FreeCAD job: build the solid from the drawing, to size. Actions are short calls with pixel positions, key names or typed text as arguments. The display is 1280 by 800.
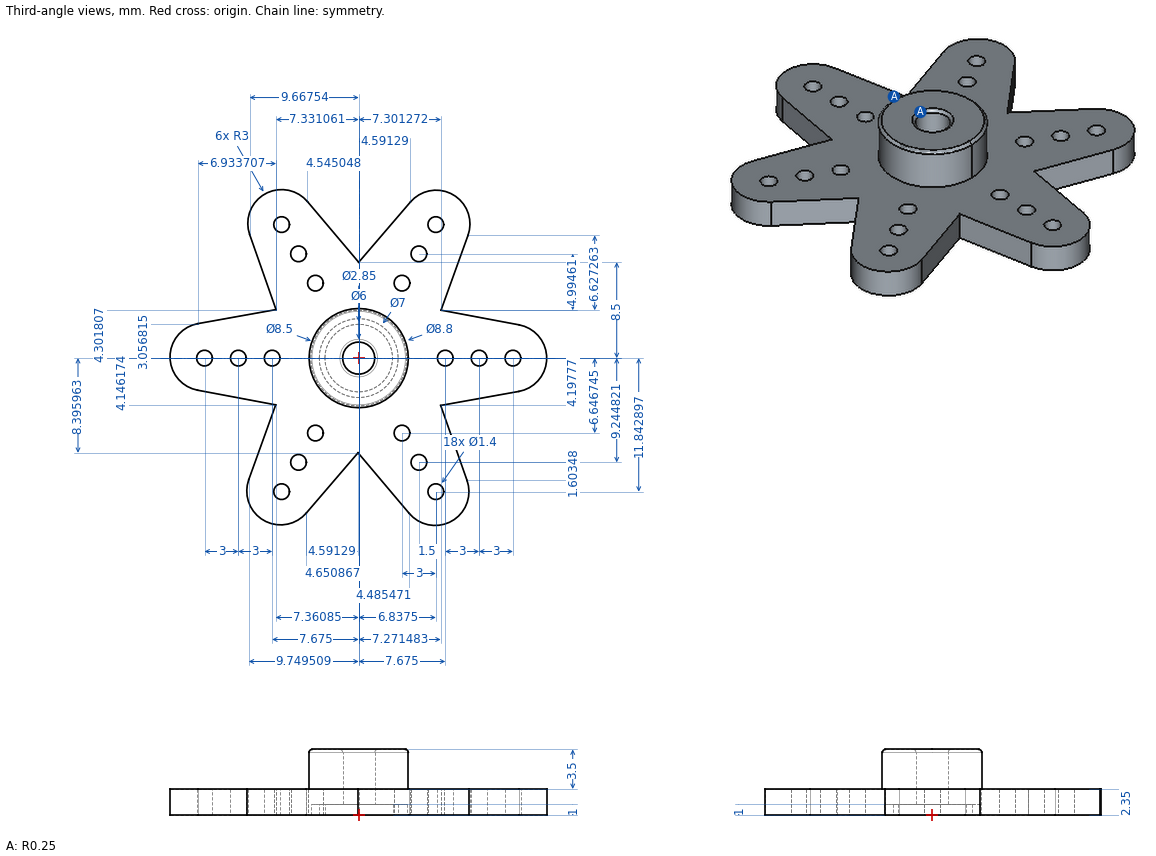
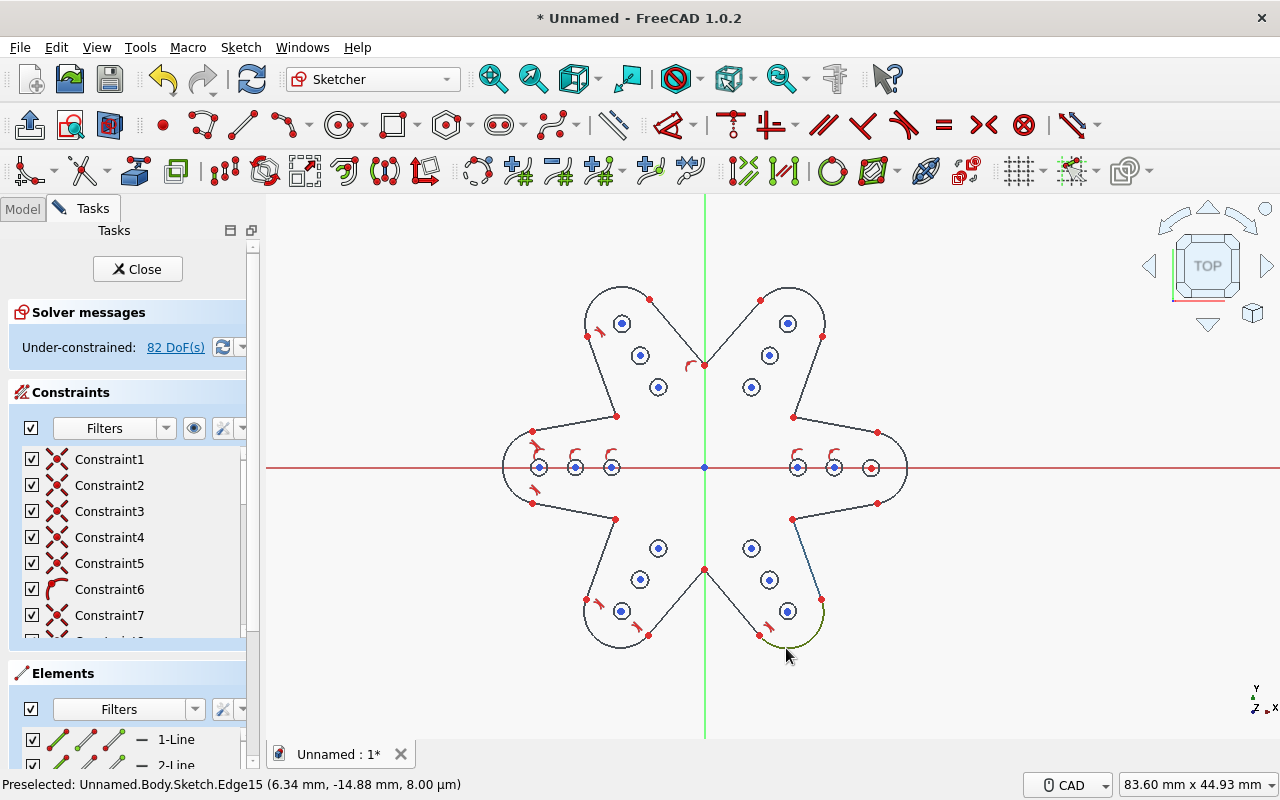
click(904, 126)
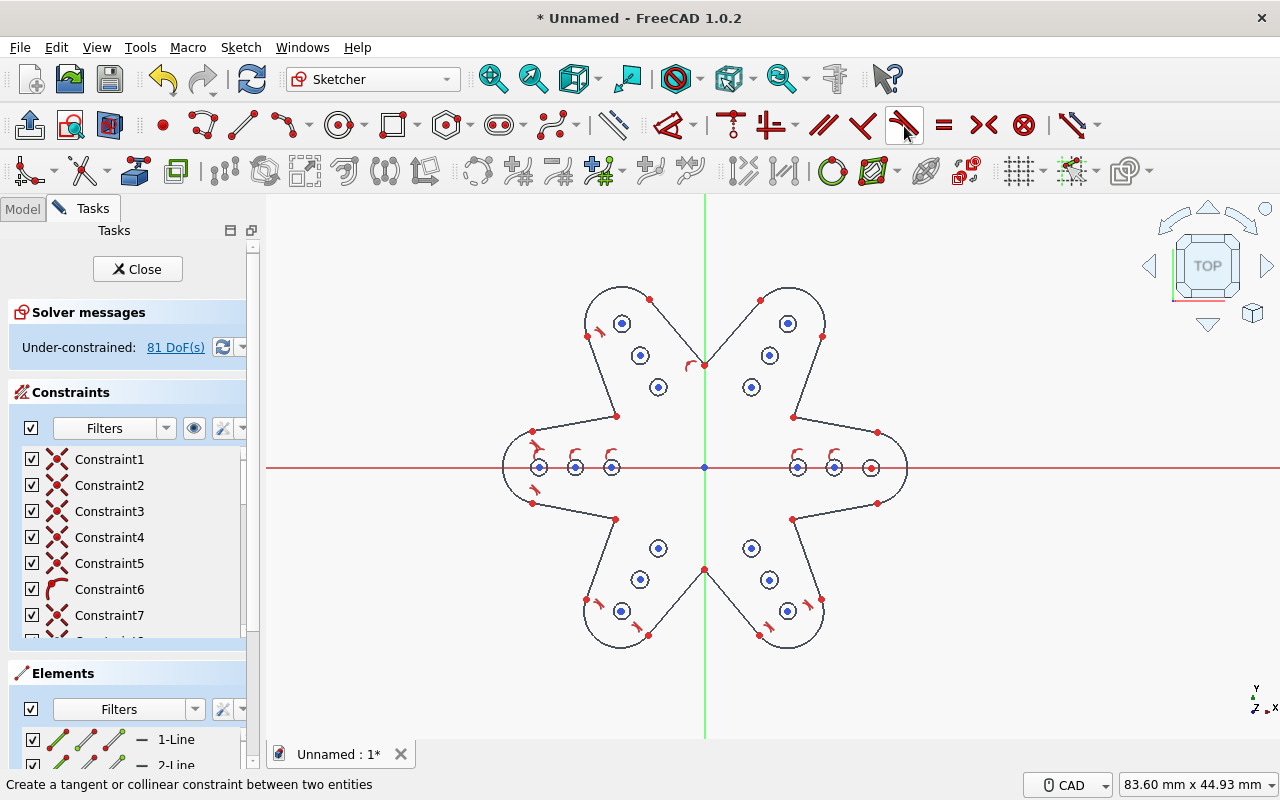
click(818, 515)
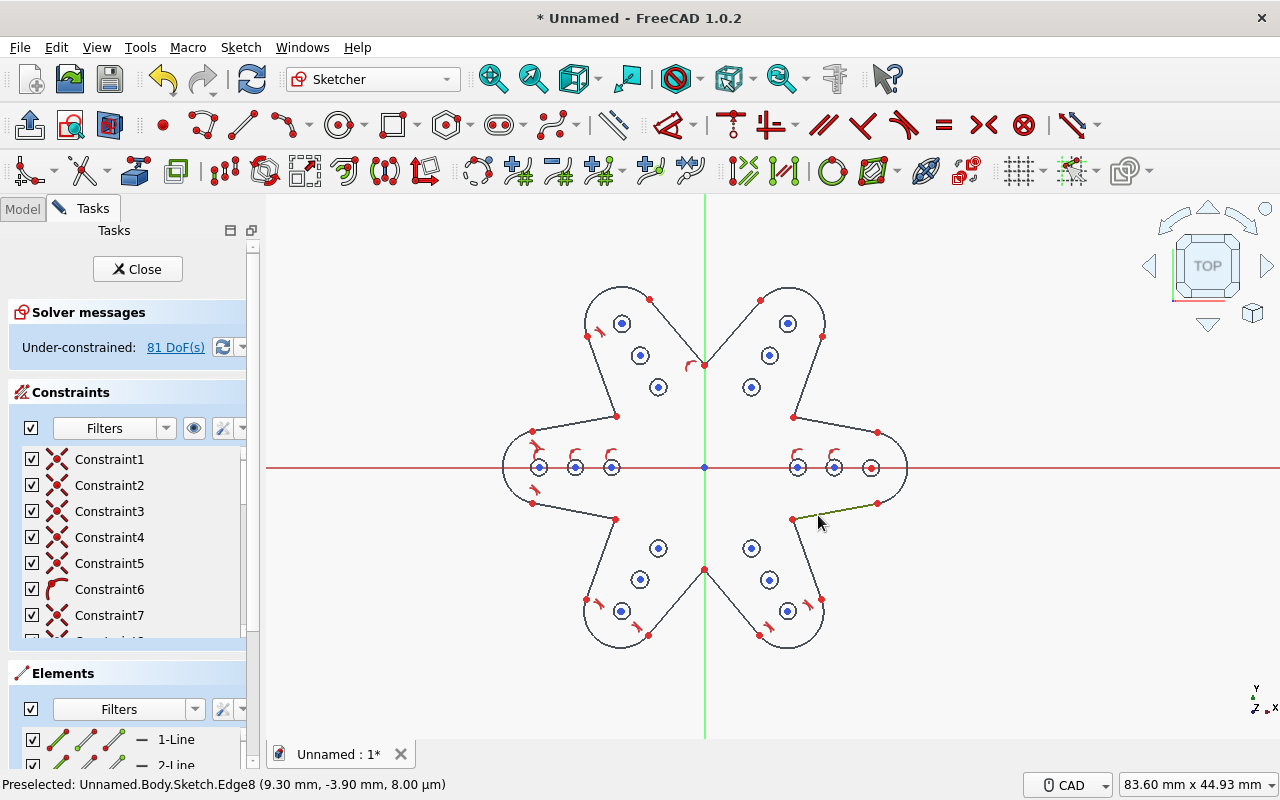
click(902, 487)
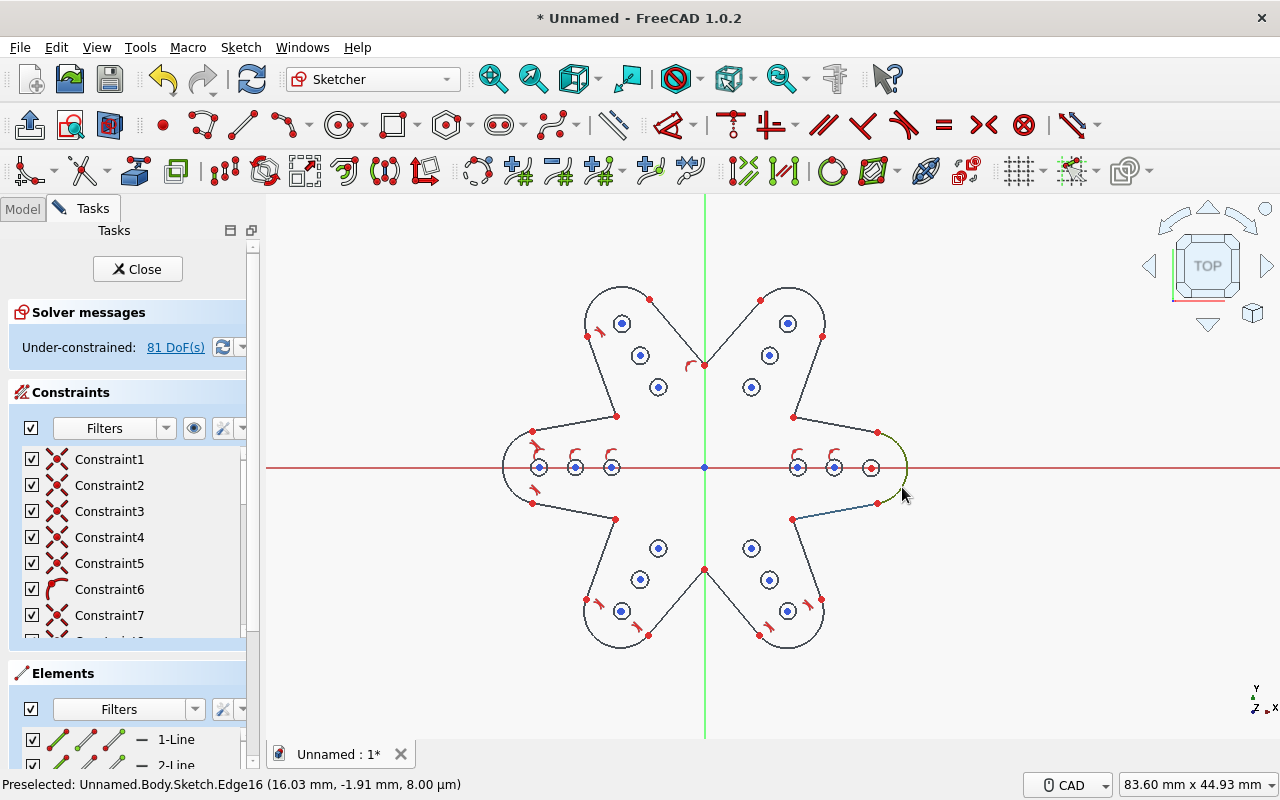
click(904, 126)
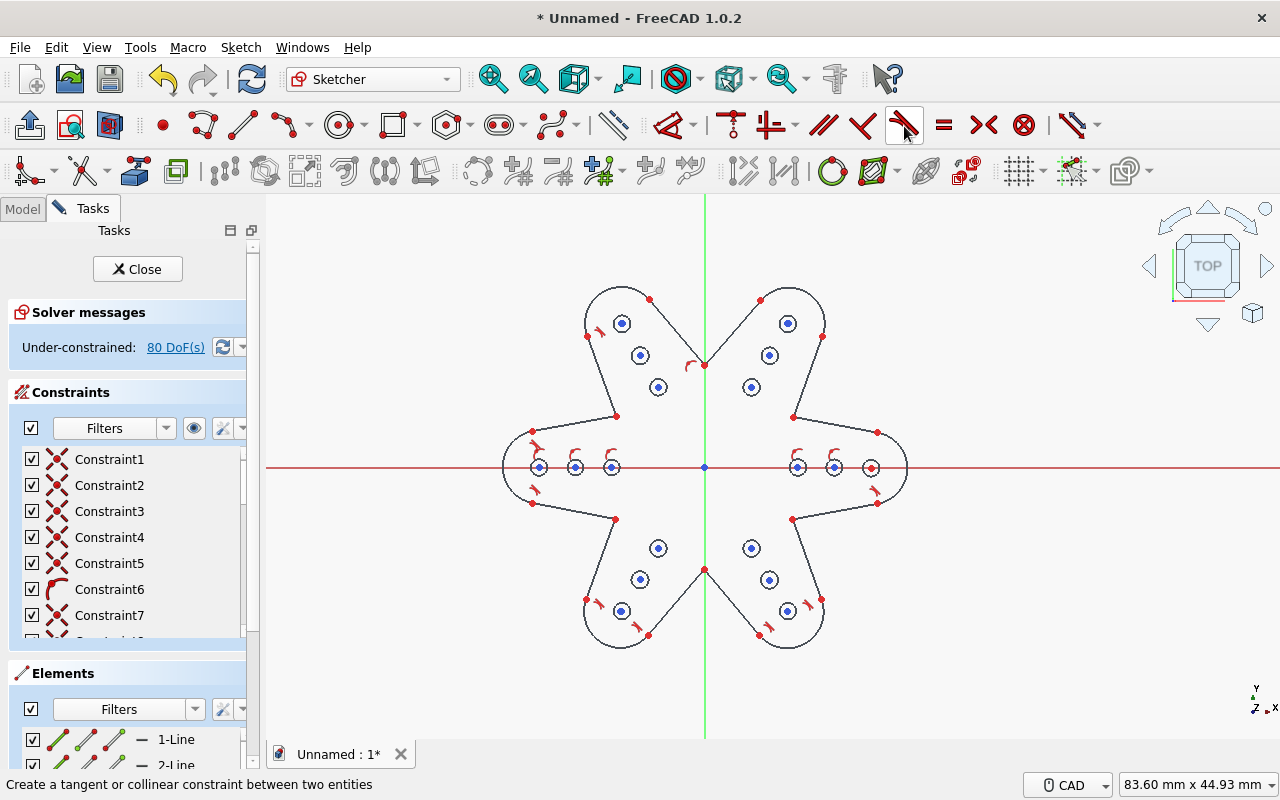
click(852, 428)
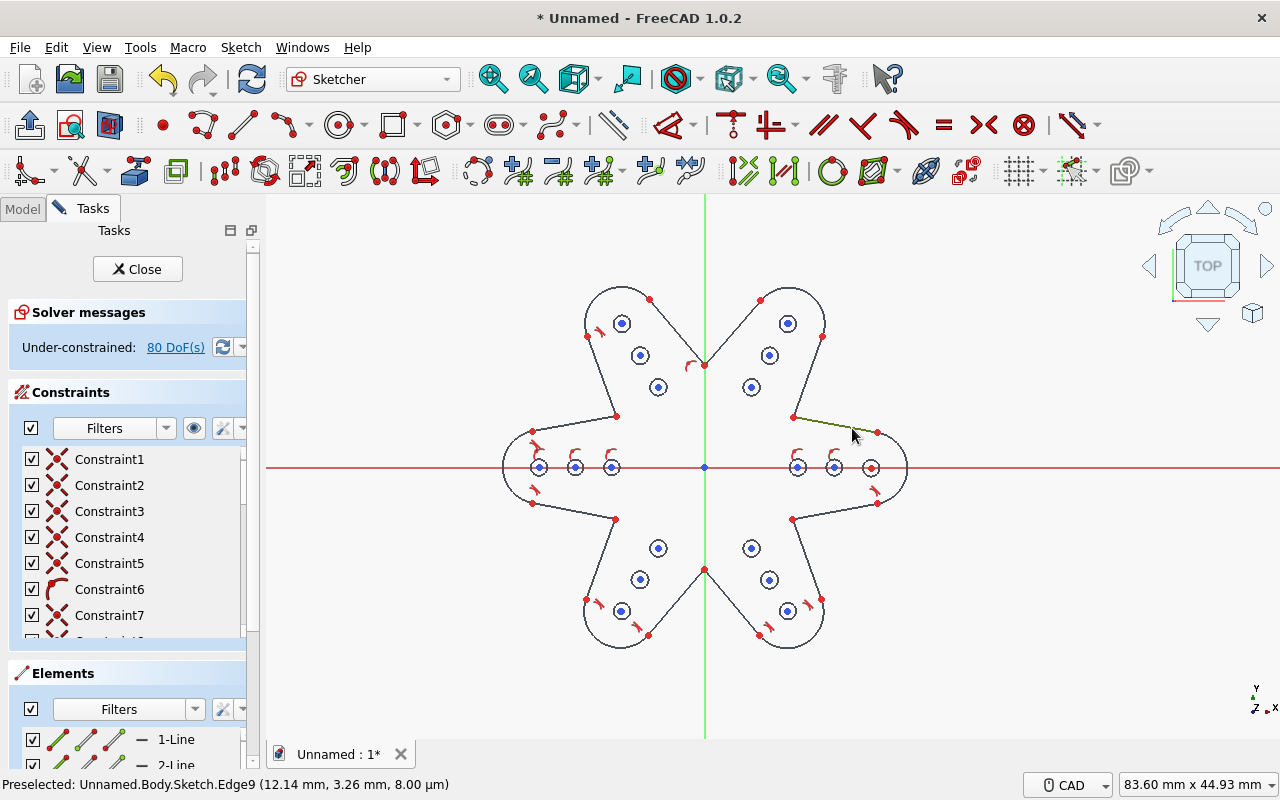
click(902, 487)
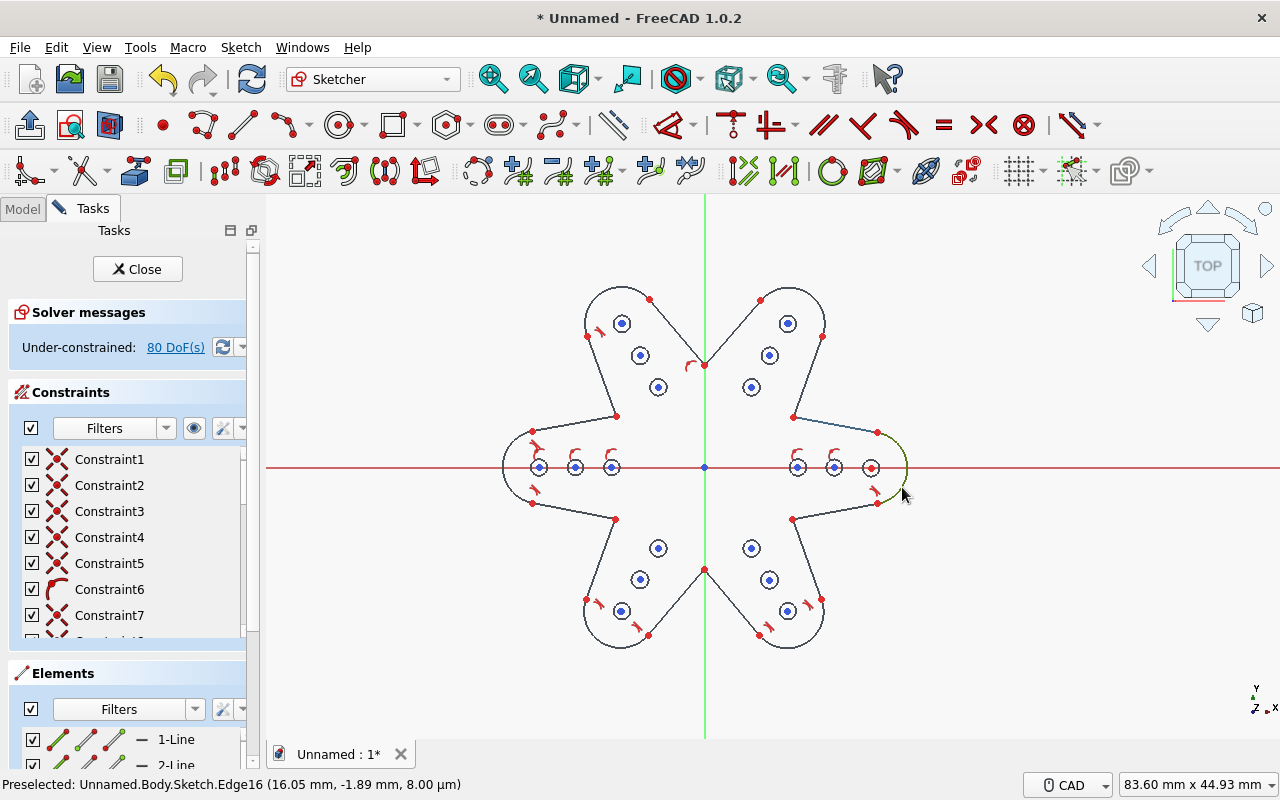
click(904, 126)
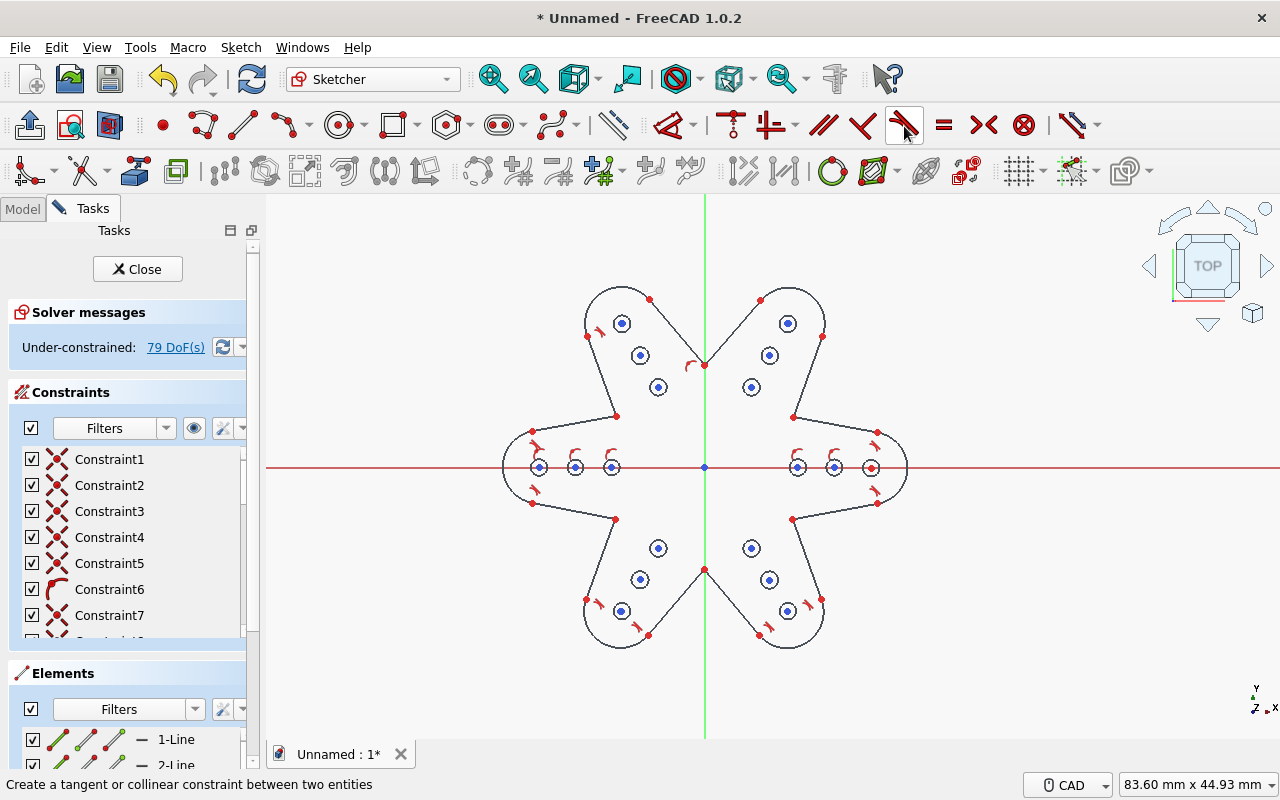
click(802, 393)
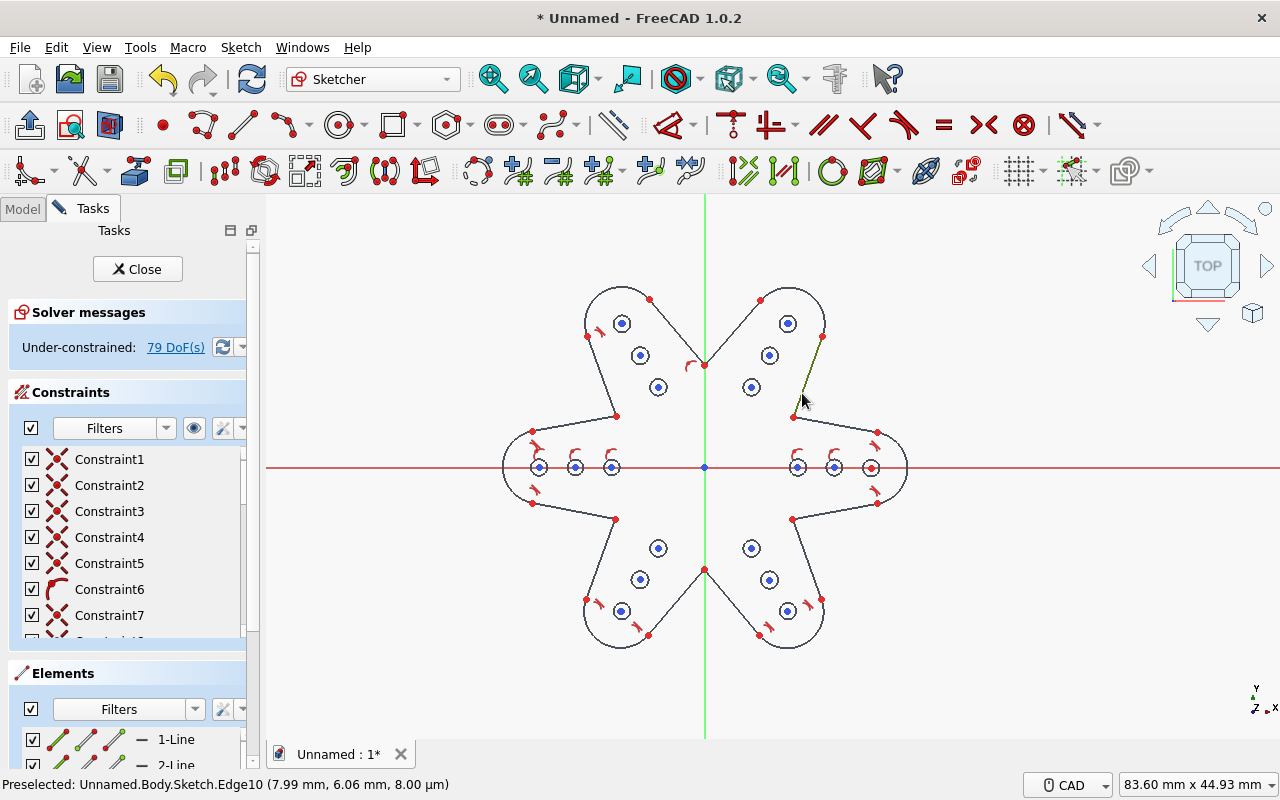
click(821, 307)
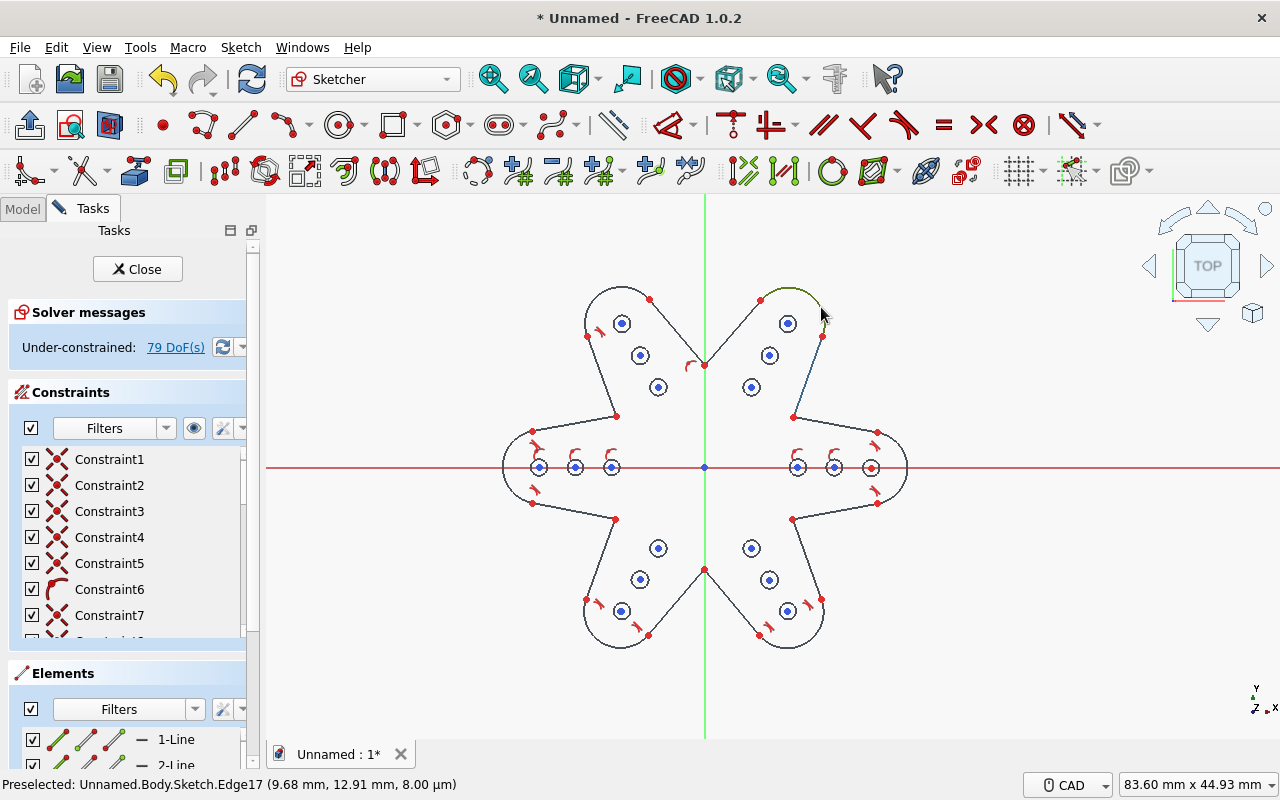
click(904, 126)